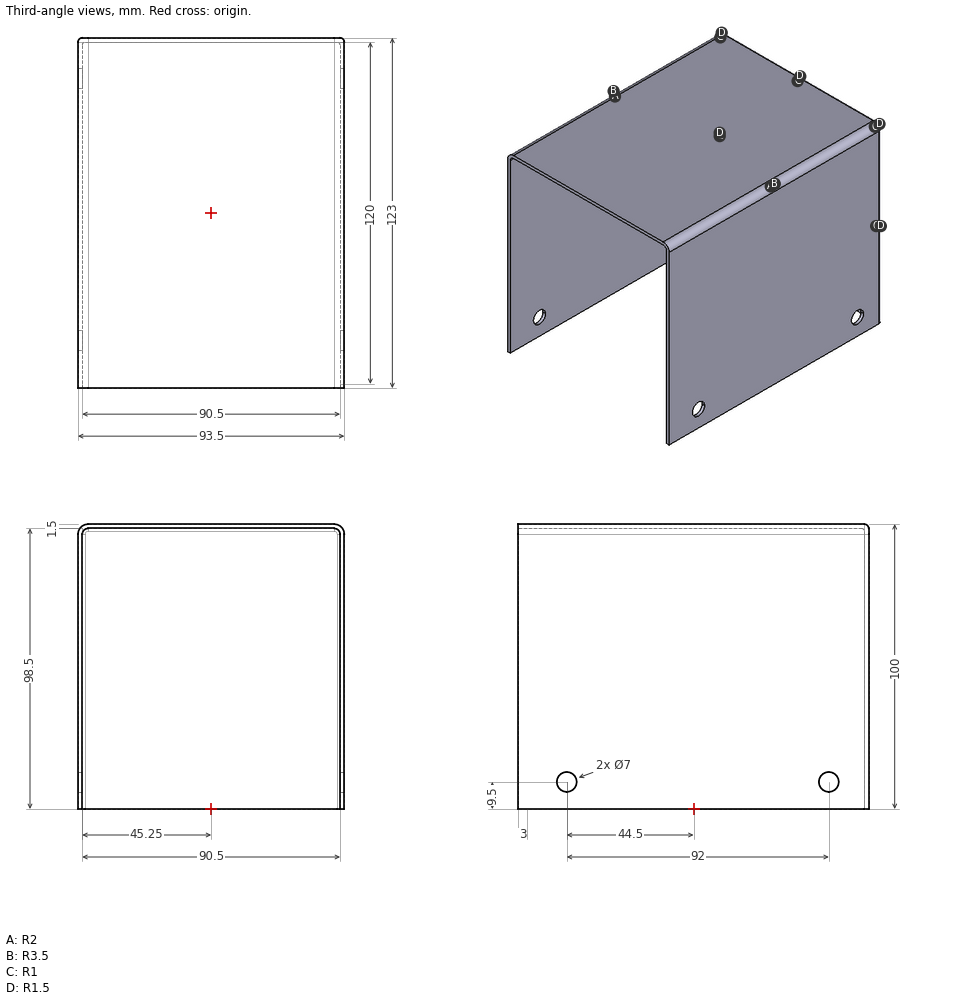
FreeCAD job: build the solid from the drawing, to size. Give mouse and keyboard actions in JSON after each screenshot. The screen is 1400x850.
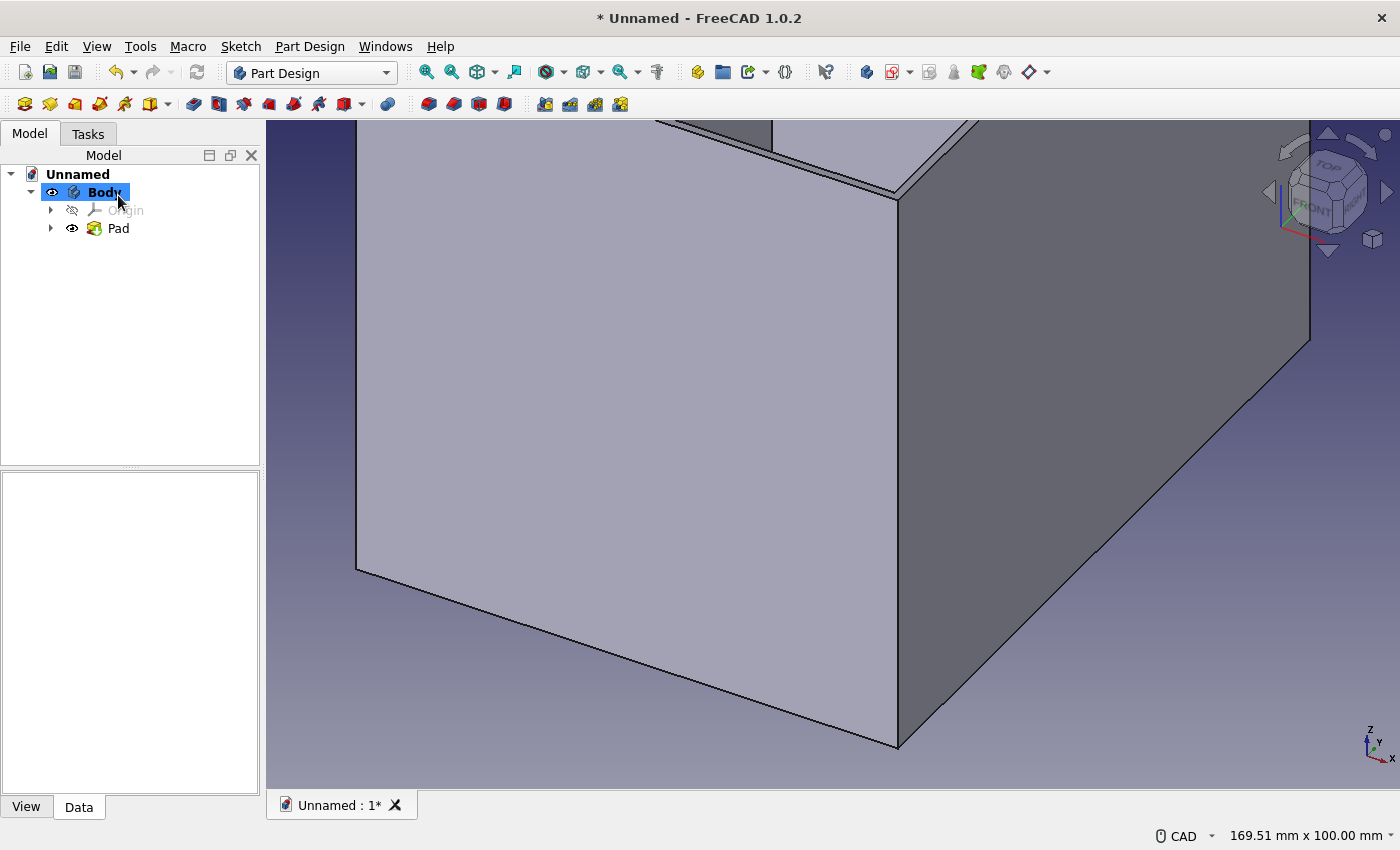
{"action": "left_click", "coordinate": [427, 72]}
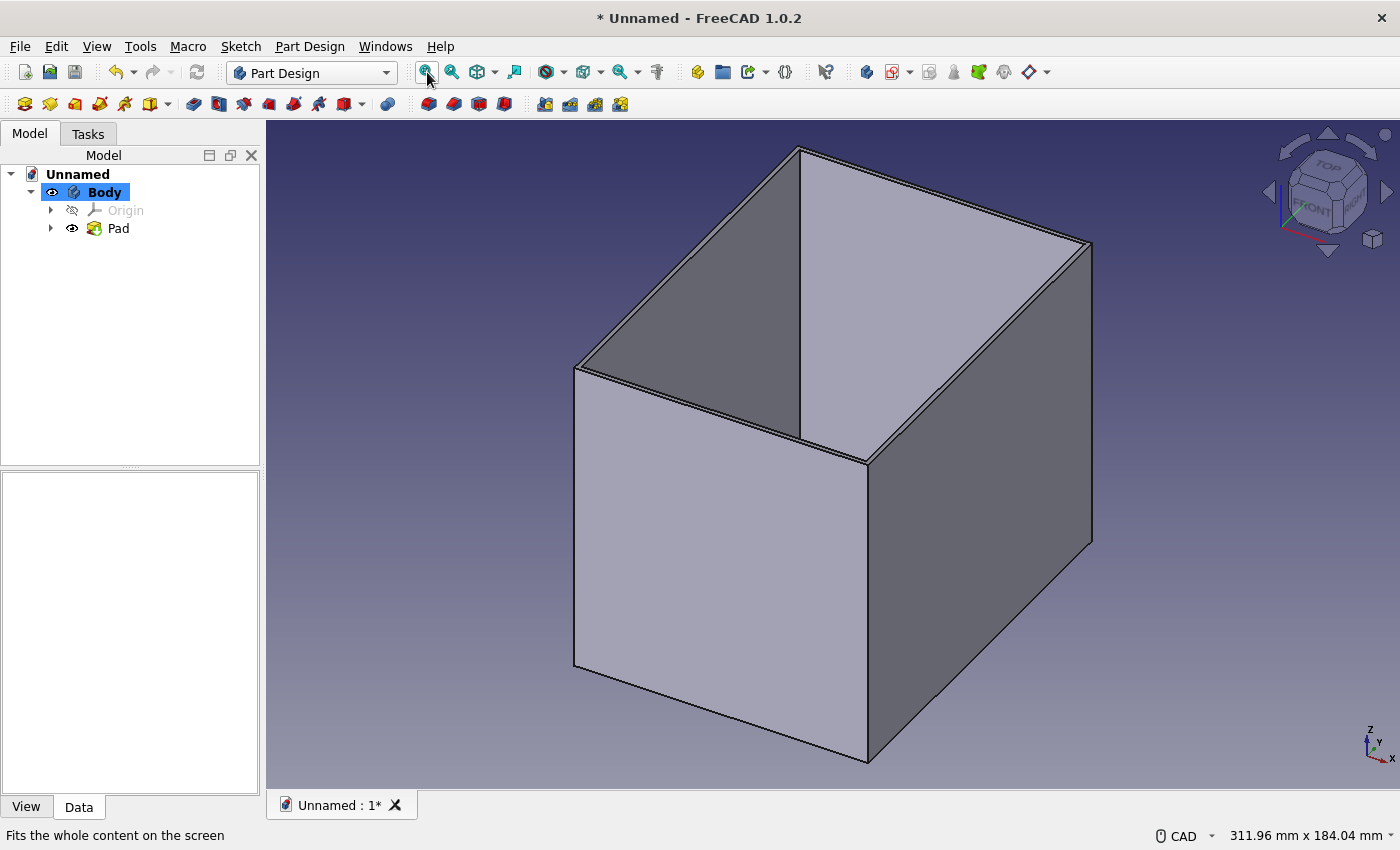
{"action": "scroll", "coordinate": [942, 389], "scroll_direction": "up", "scroll_amount": 10}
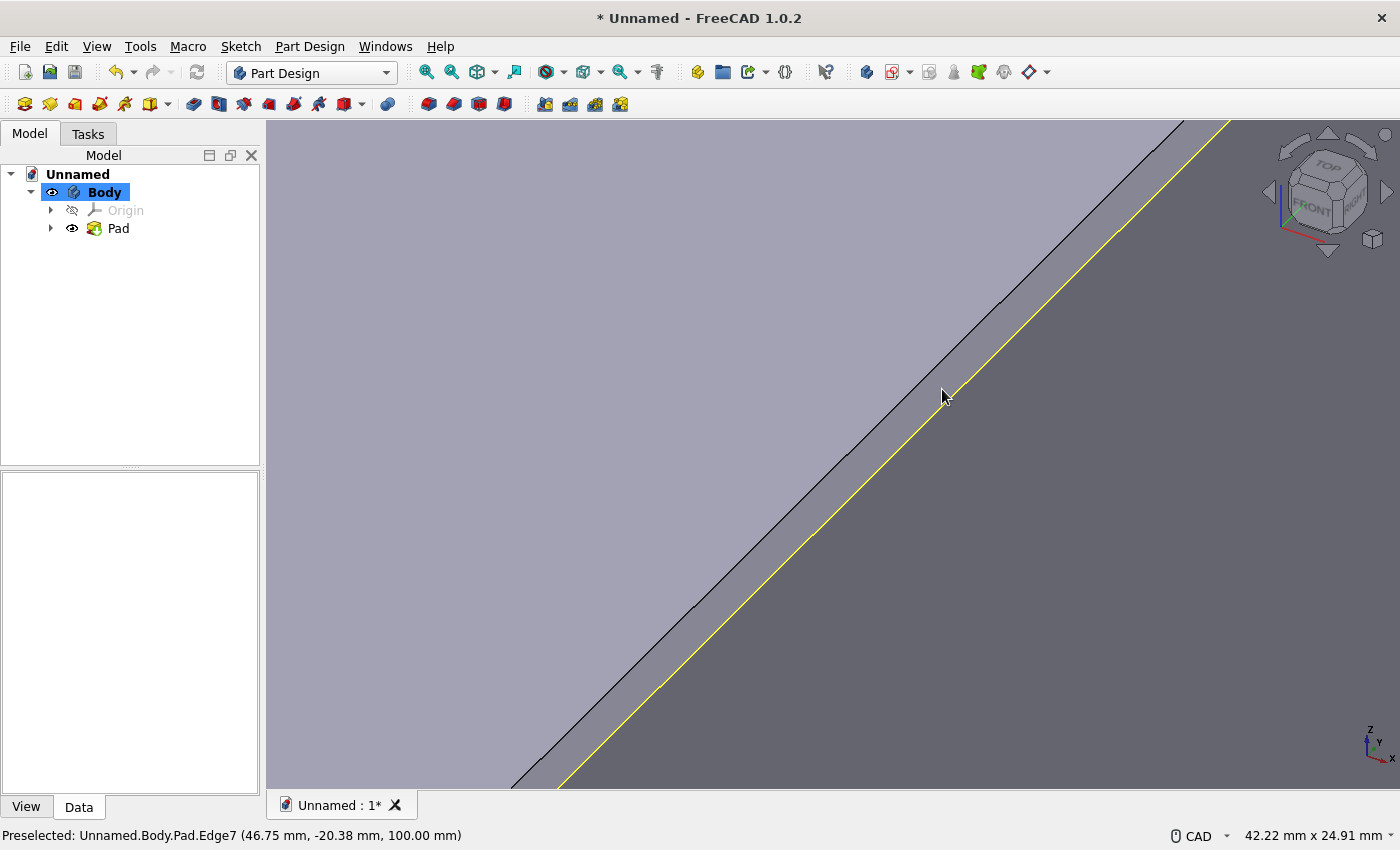
{"action": "left_click", "coordinate": [940, 392]}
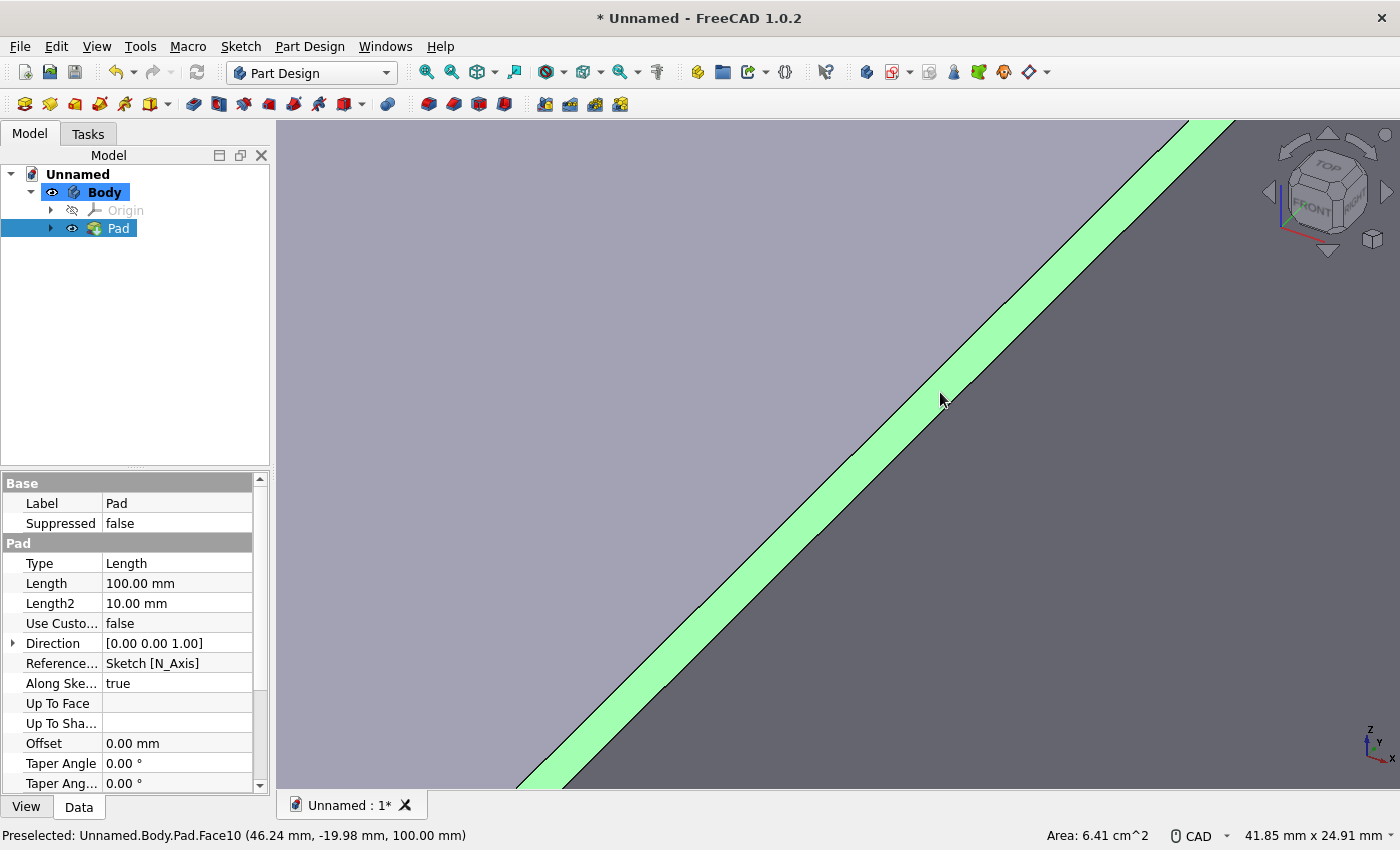
{"action": "left_click", "coordinate": [892, 72]}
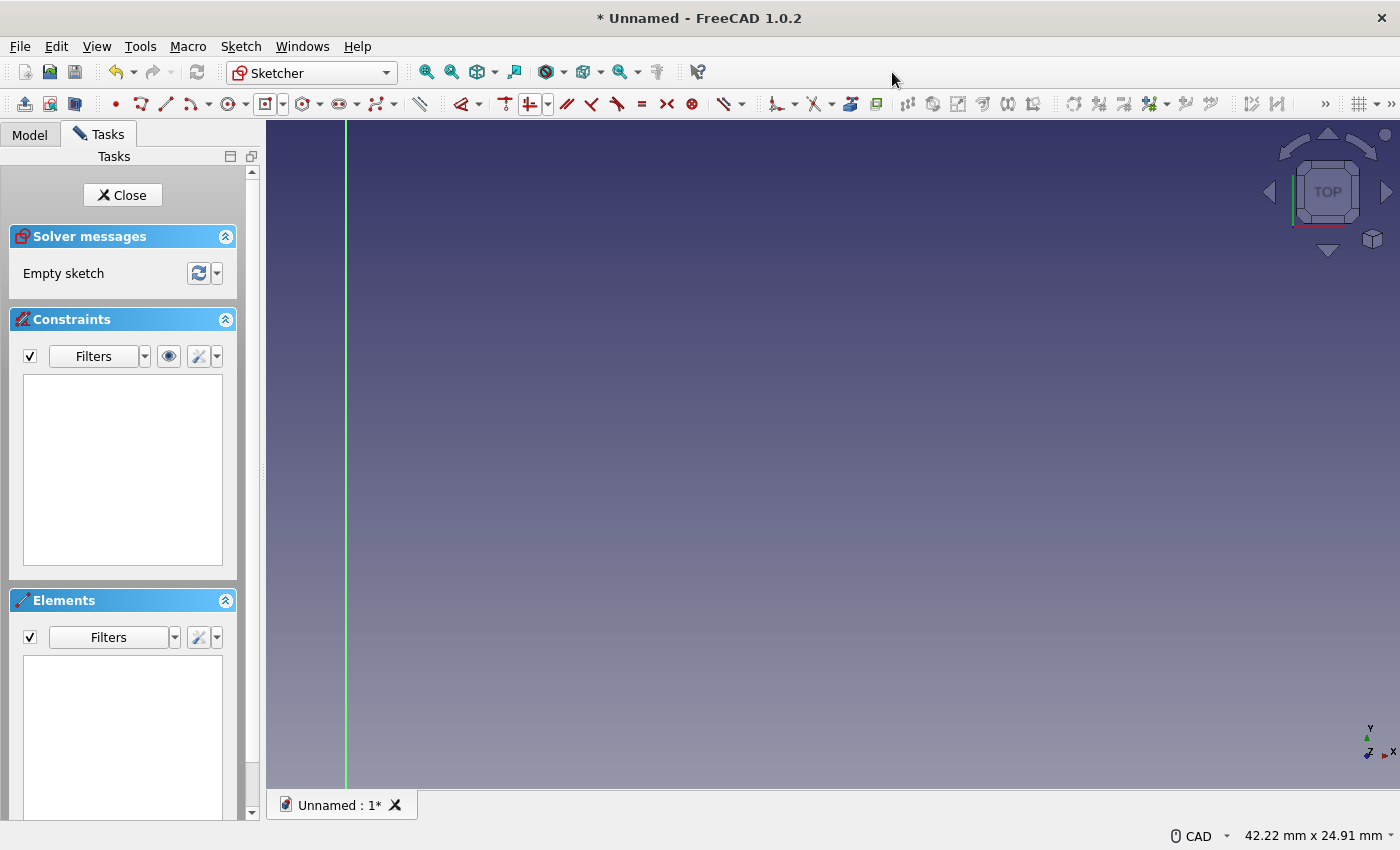
{"action": "scroll", "coordinate": [830, 367], "scroll_direction": "down", "scroll_amount": 10}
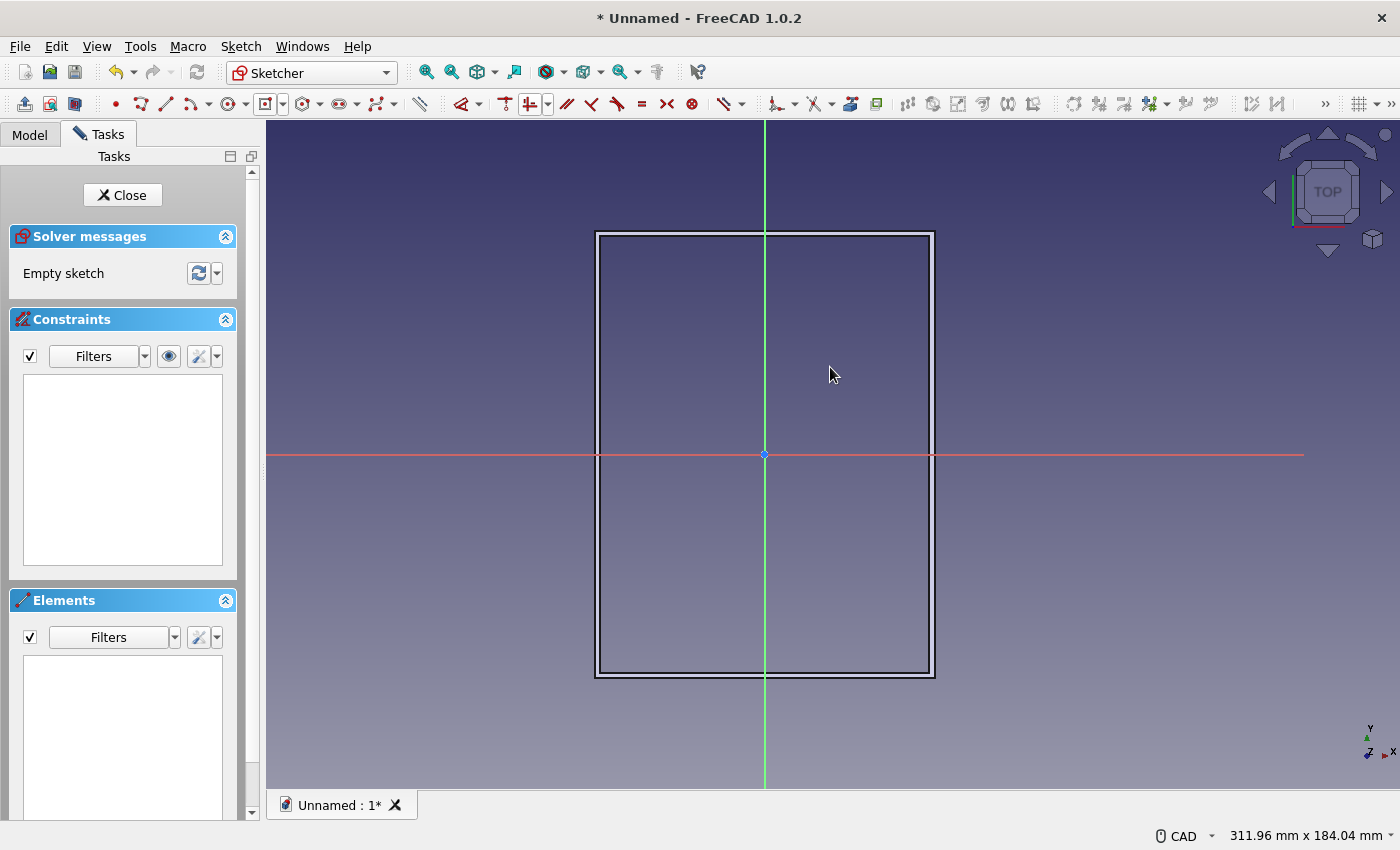
{"action": "left_click", "coordinate": [264, 104]}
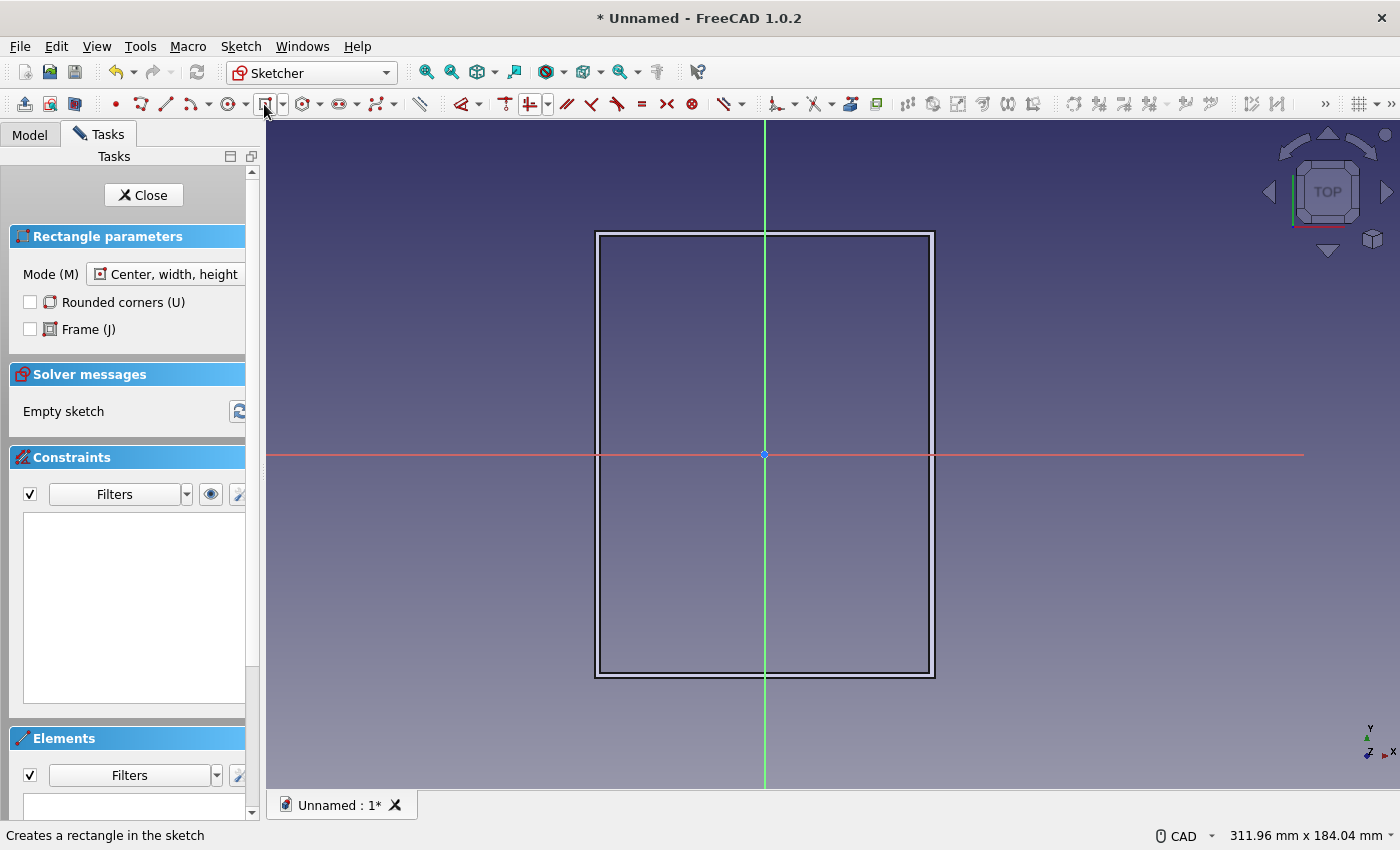
{"action": "left_click", "coordinate": [765, 455]}
{"action": "mouse_move", "coordinate": [935, 231]}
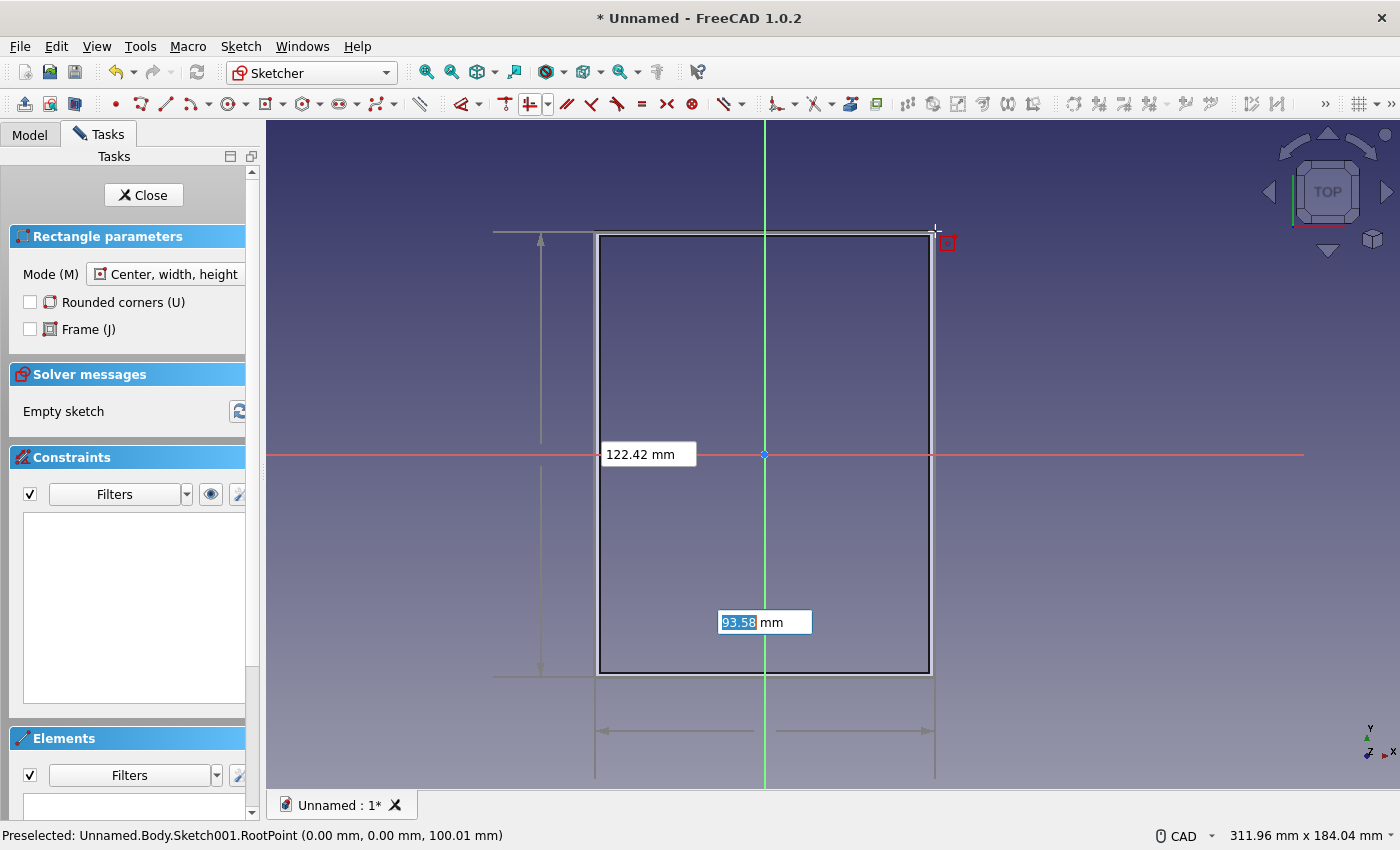
{"action": "type", "text": "93.5"}
{"action": "key", "text": "Tab"}
{"action": "type", "text": "123"}
{"action": "key", "text": "Return"}
{"action": "key", "text": "Escape"}